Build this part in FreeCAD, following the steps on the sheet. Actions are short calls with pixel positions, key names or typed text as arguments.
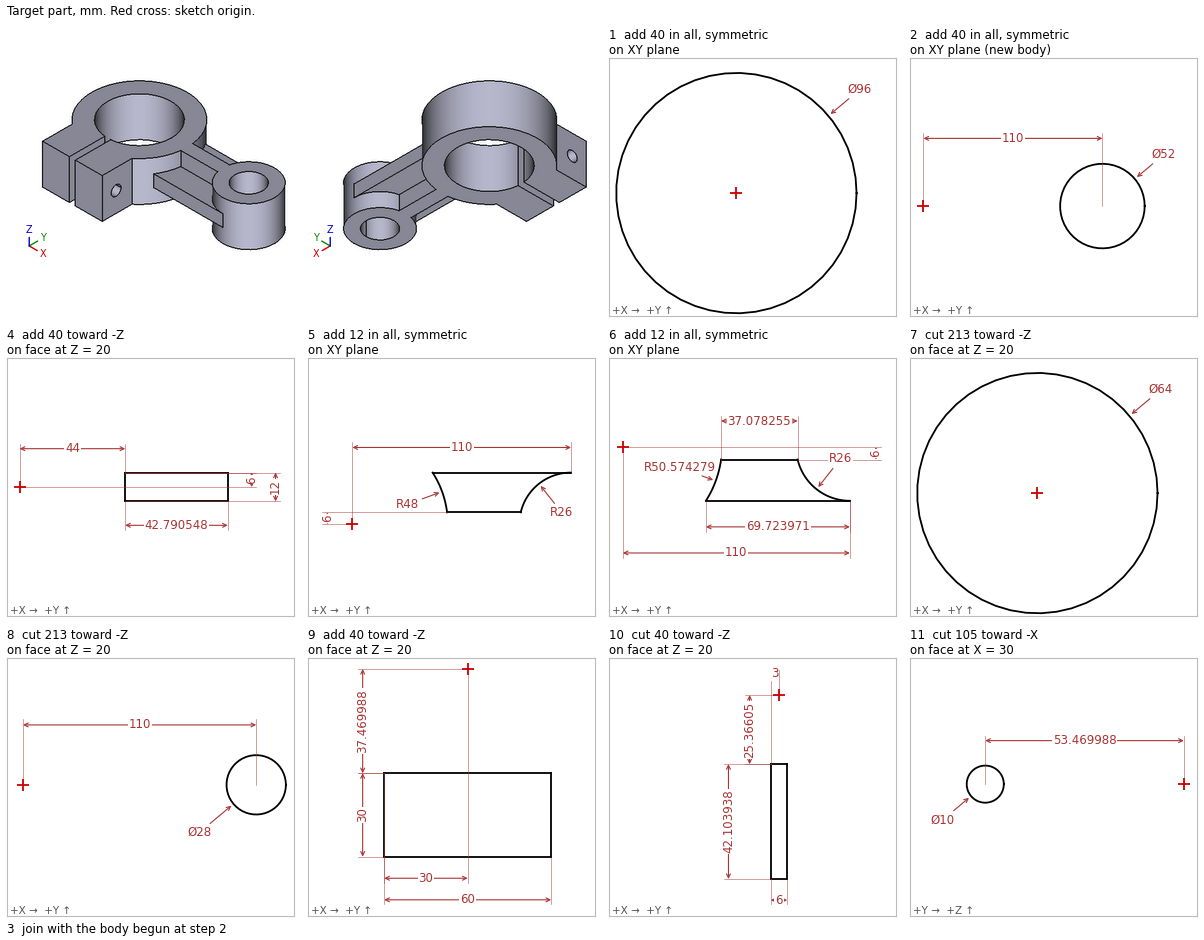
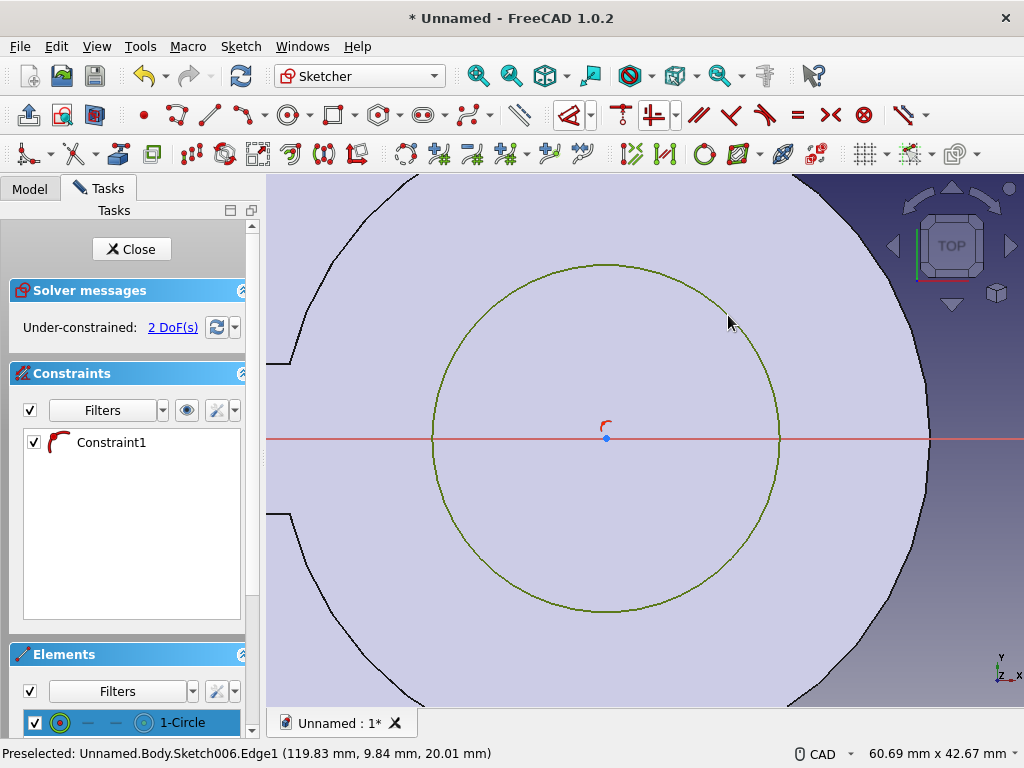
click(590, 116)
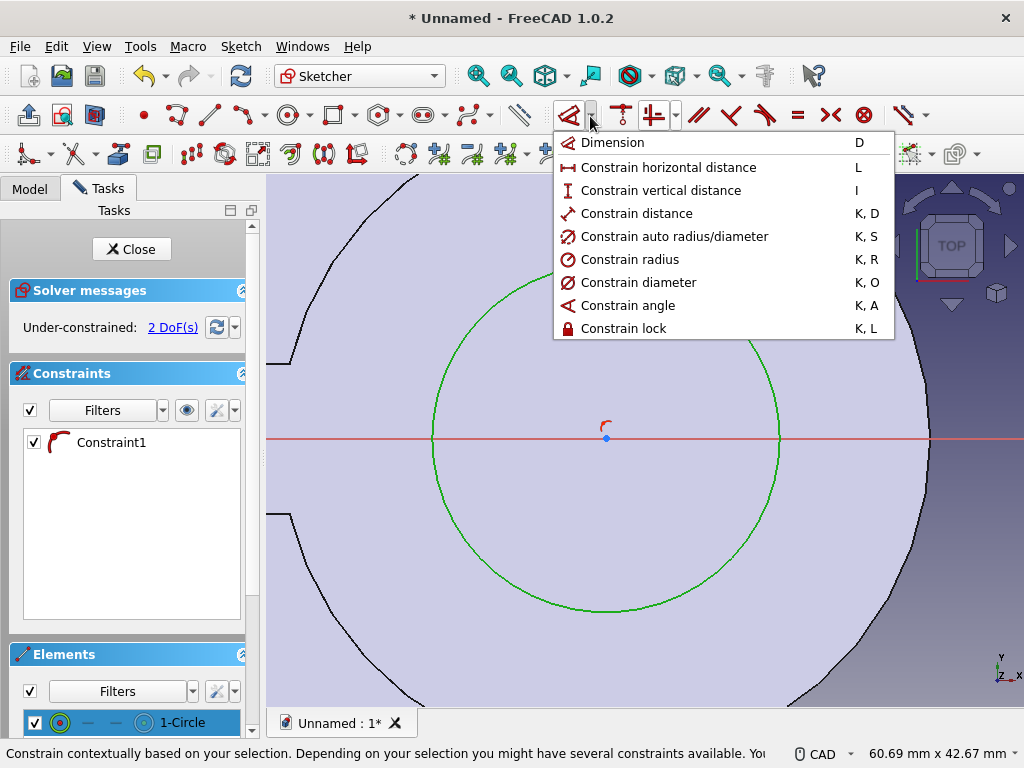
click(724, 282)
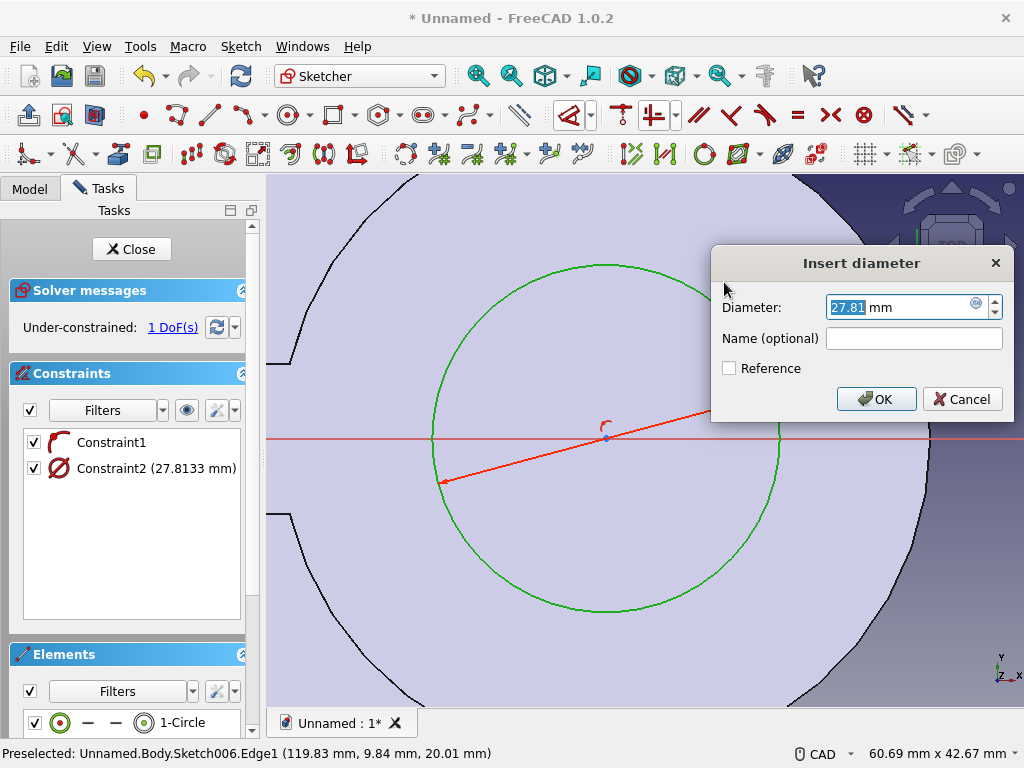
text(28)
key(Return)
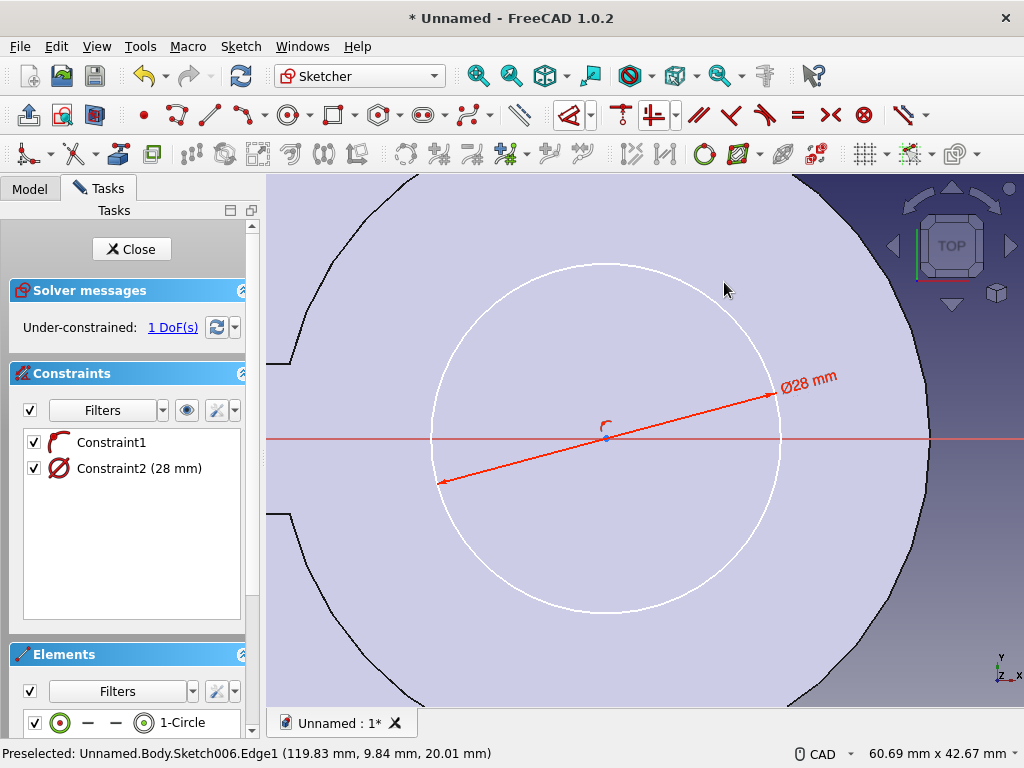
click(606, 439)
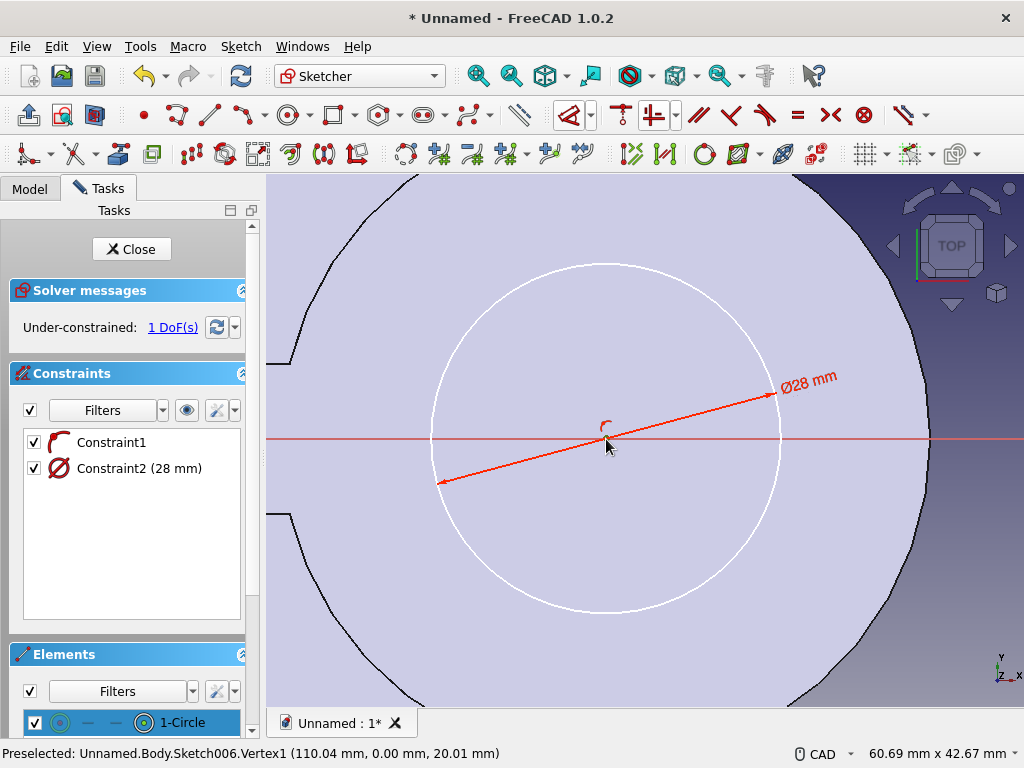
click(590, 116)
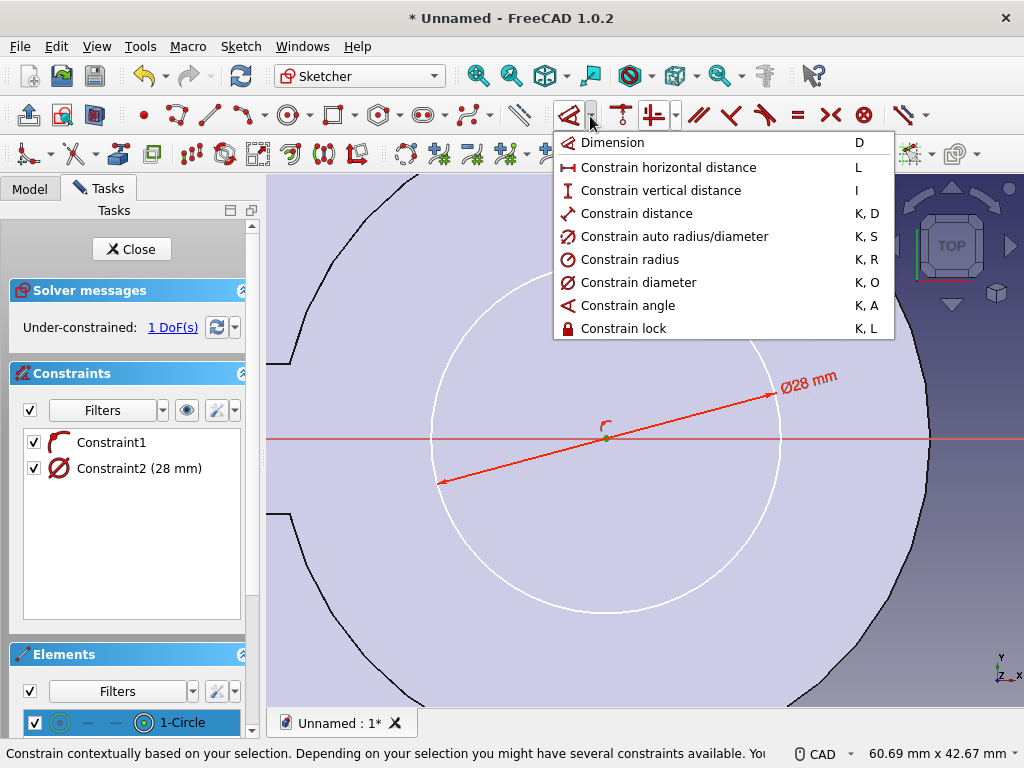
click(724, 168)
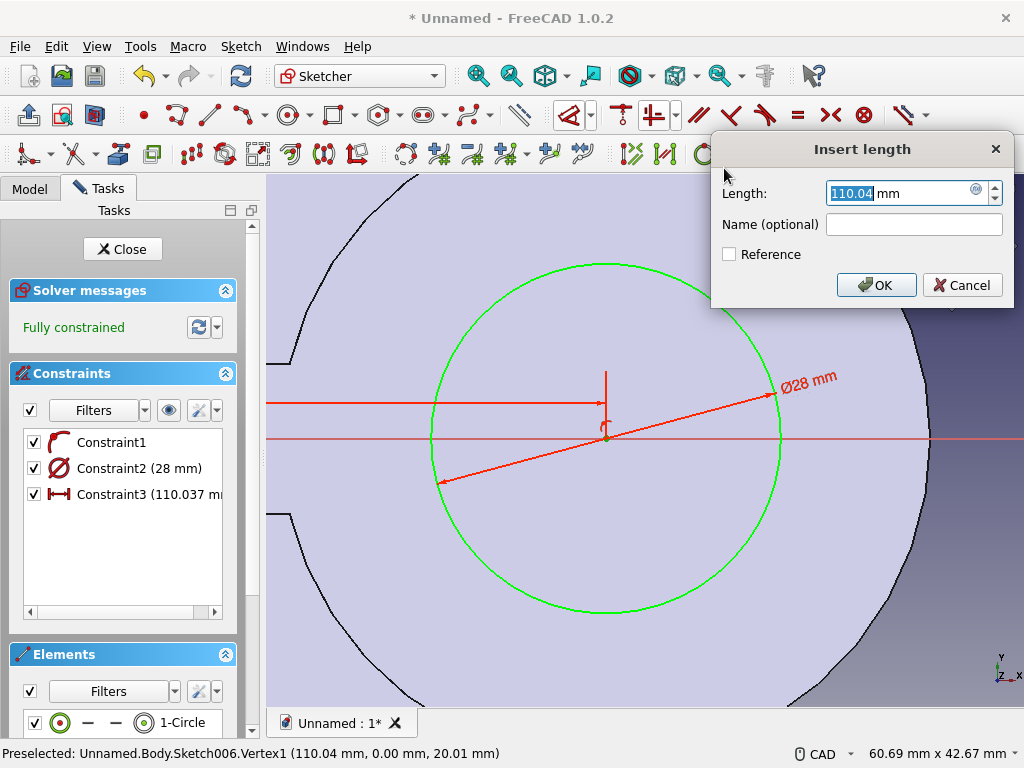
text(110)
key(Return)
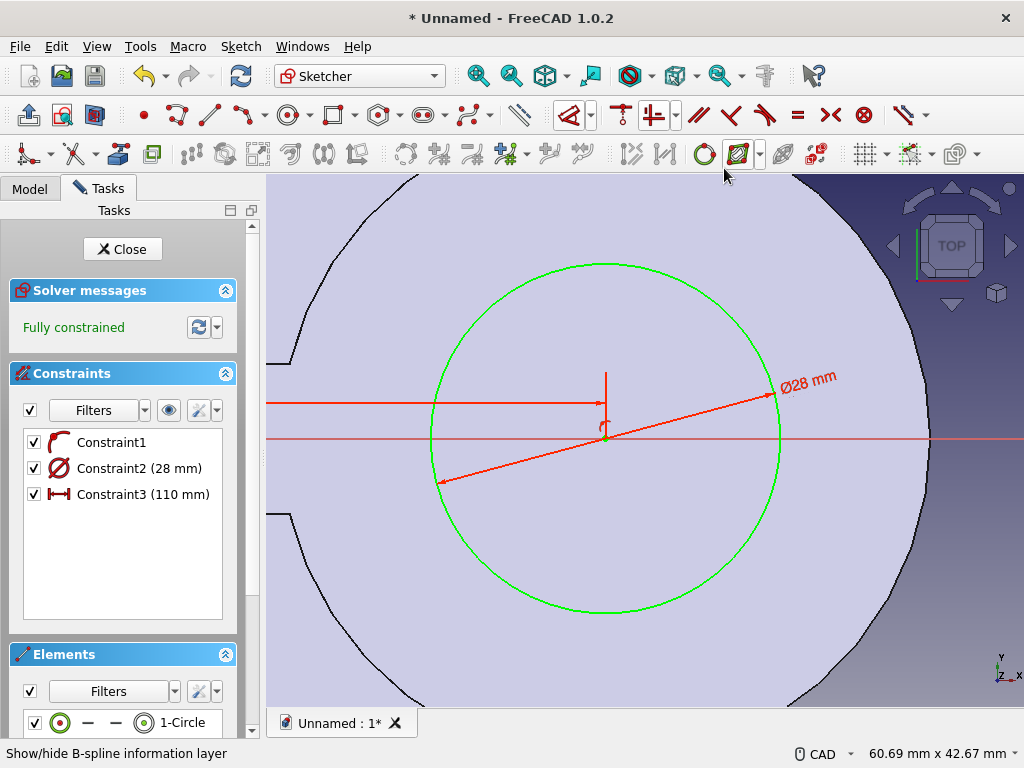
click(123, 249)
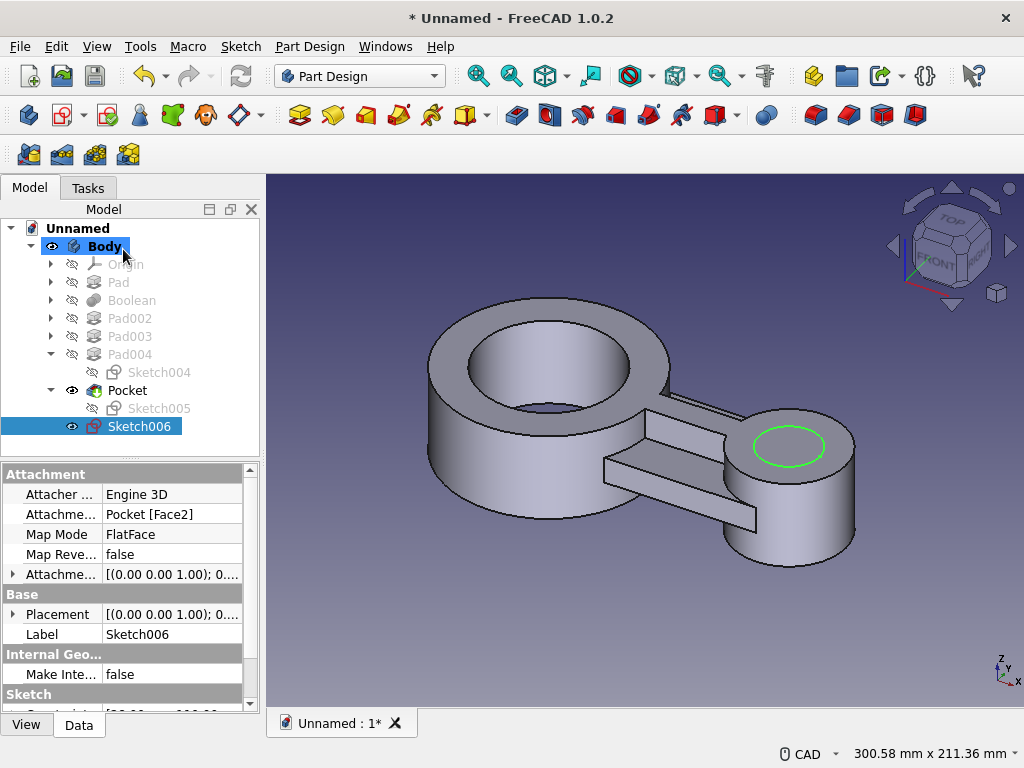
click(517, 116)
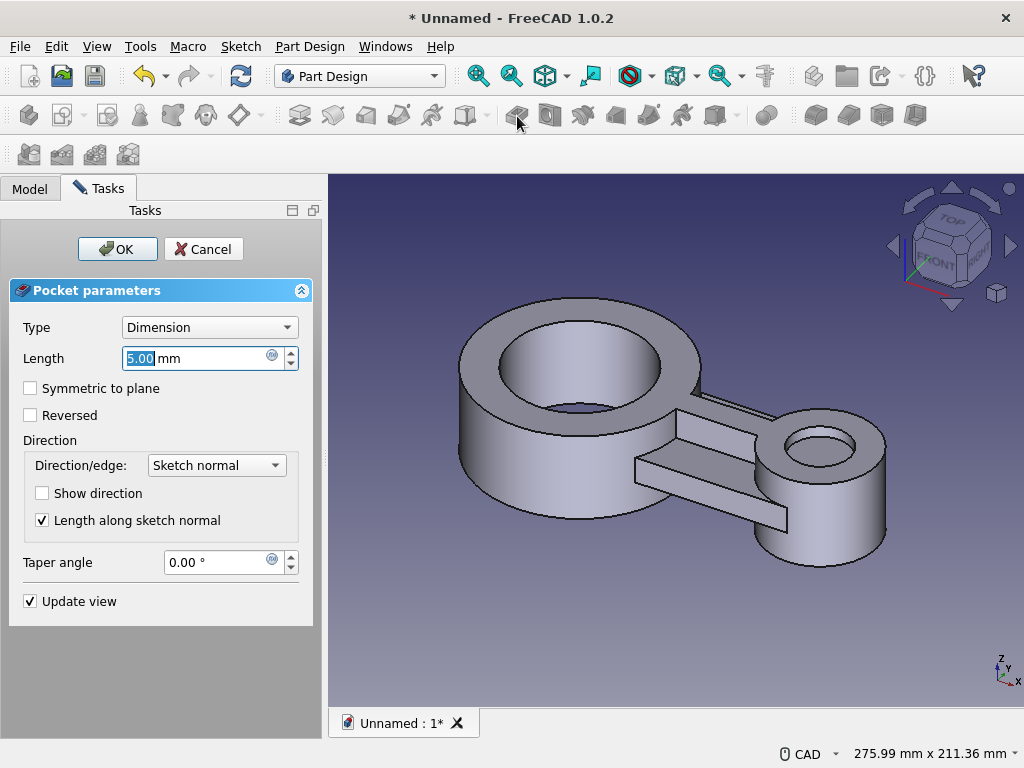
text(213)
key(Tab)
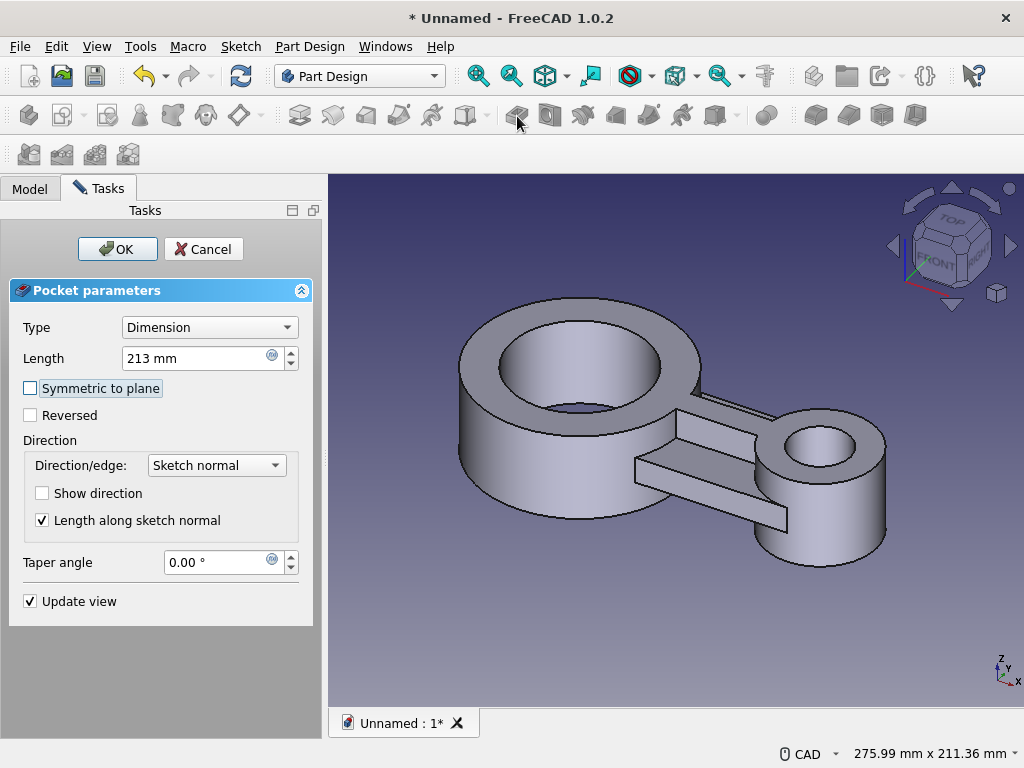
click(118, 249)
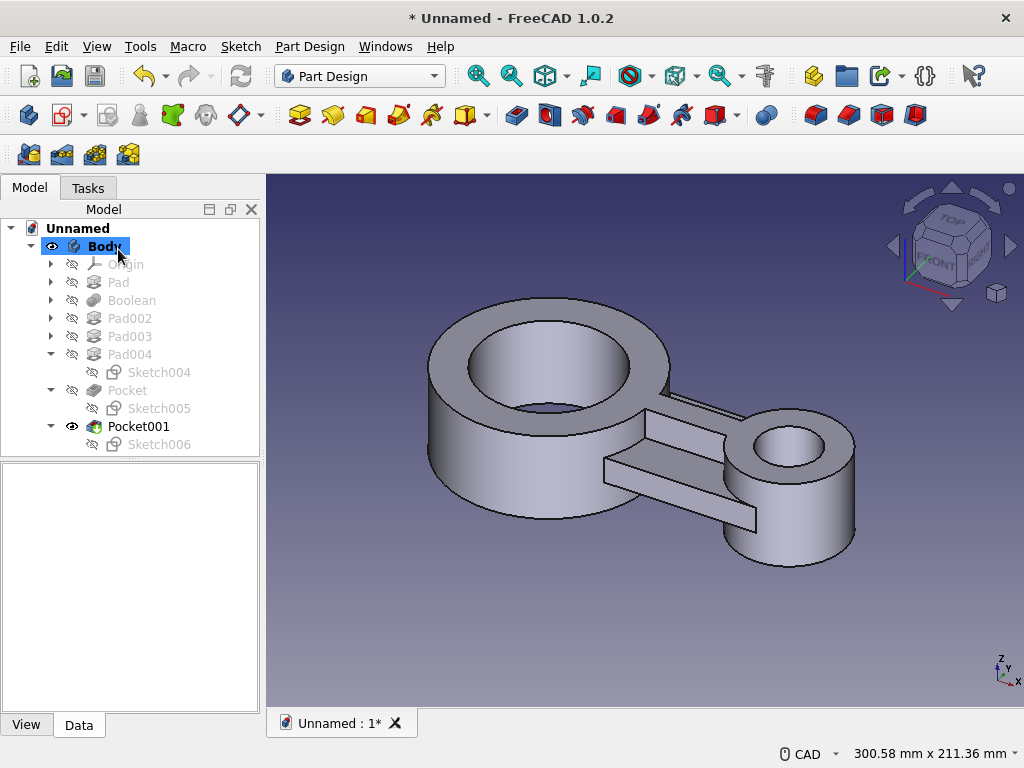
click(645, 398)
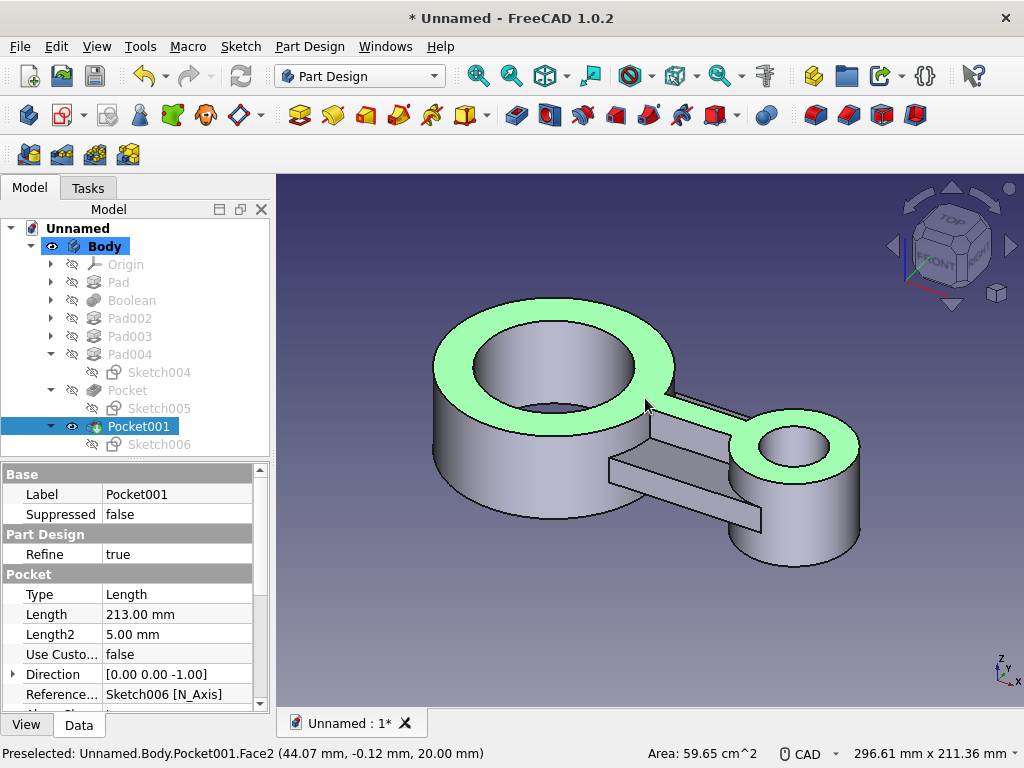
click(62, 116)